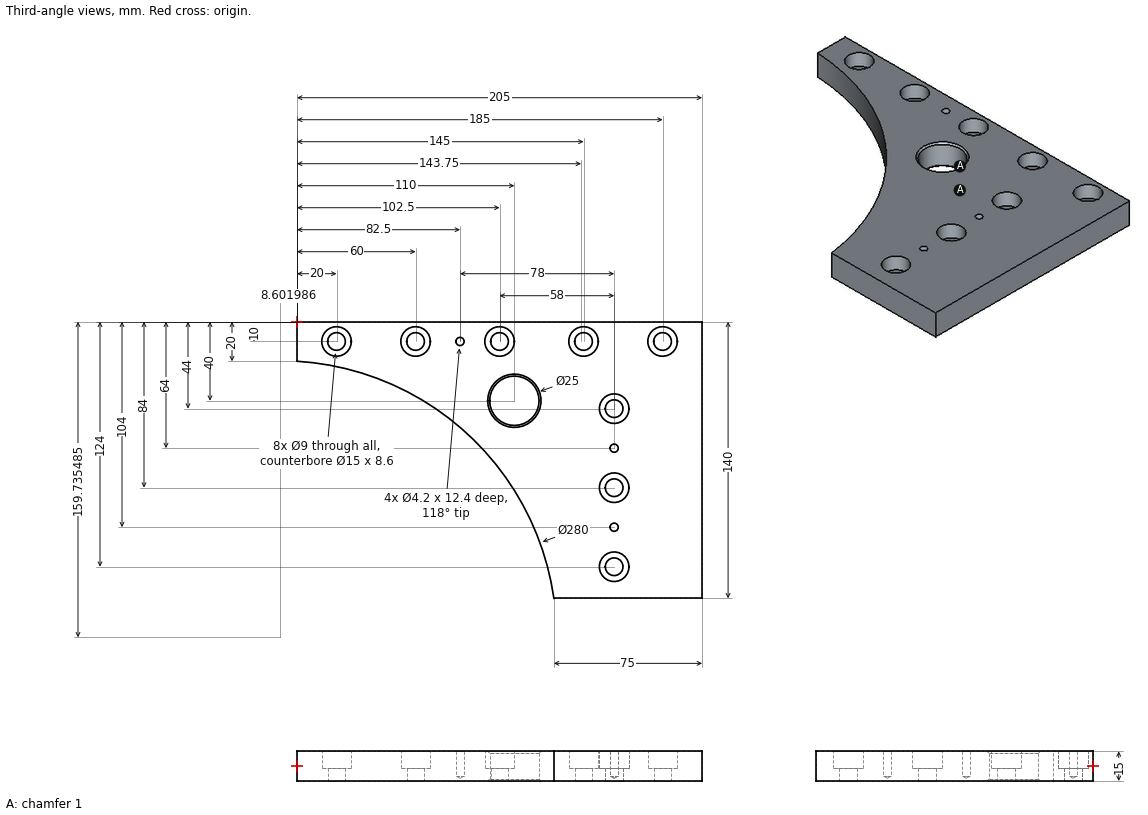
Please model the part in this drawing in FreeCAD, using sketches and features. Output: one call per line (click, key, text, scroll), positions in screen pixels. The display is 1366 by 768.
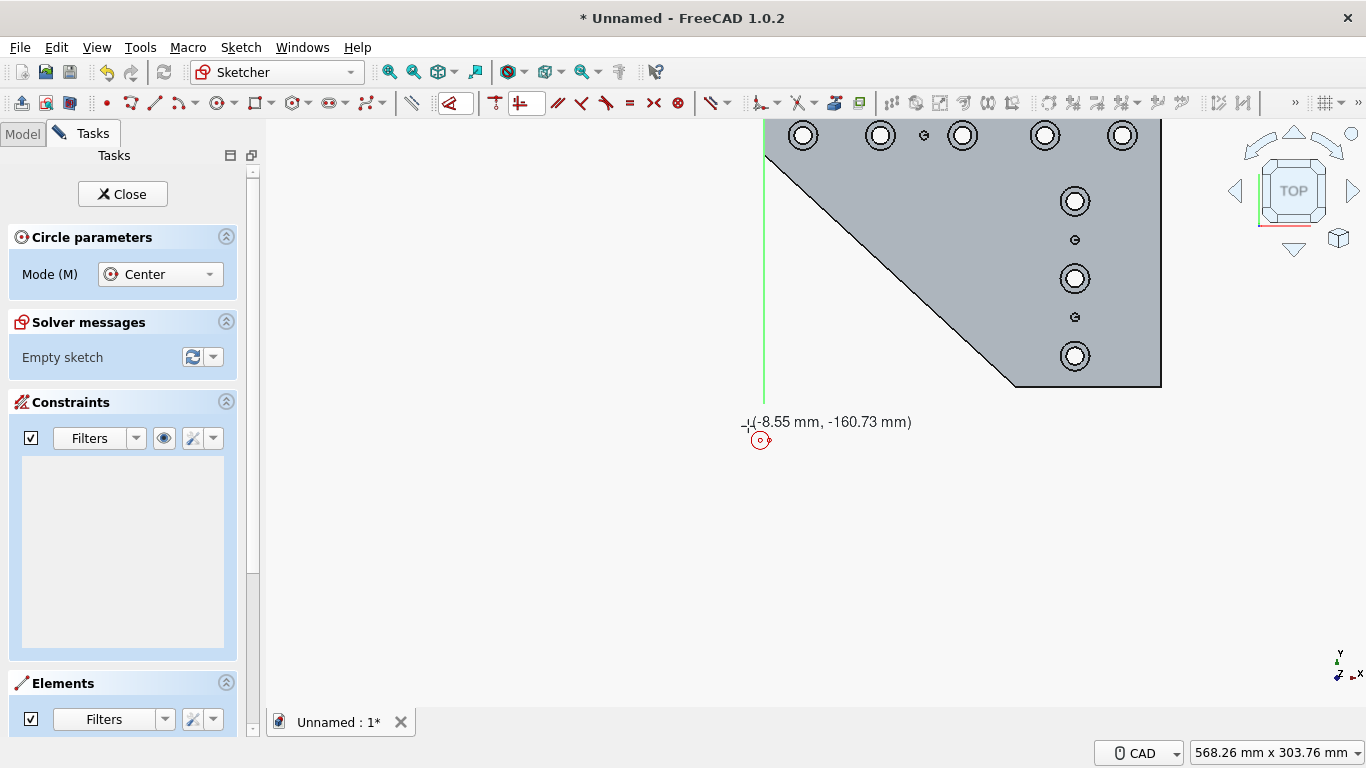
click(748, 425)
click(939, 234)
key(Escape)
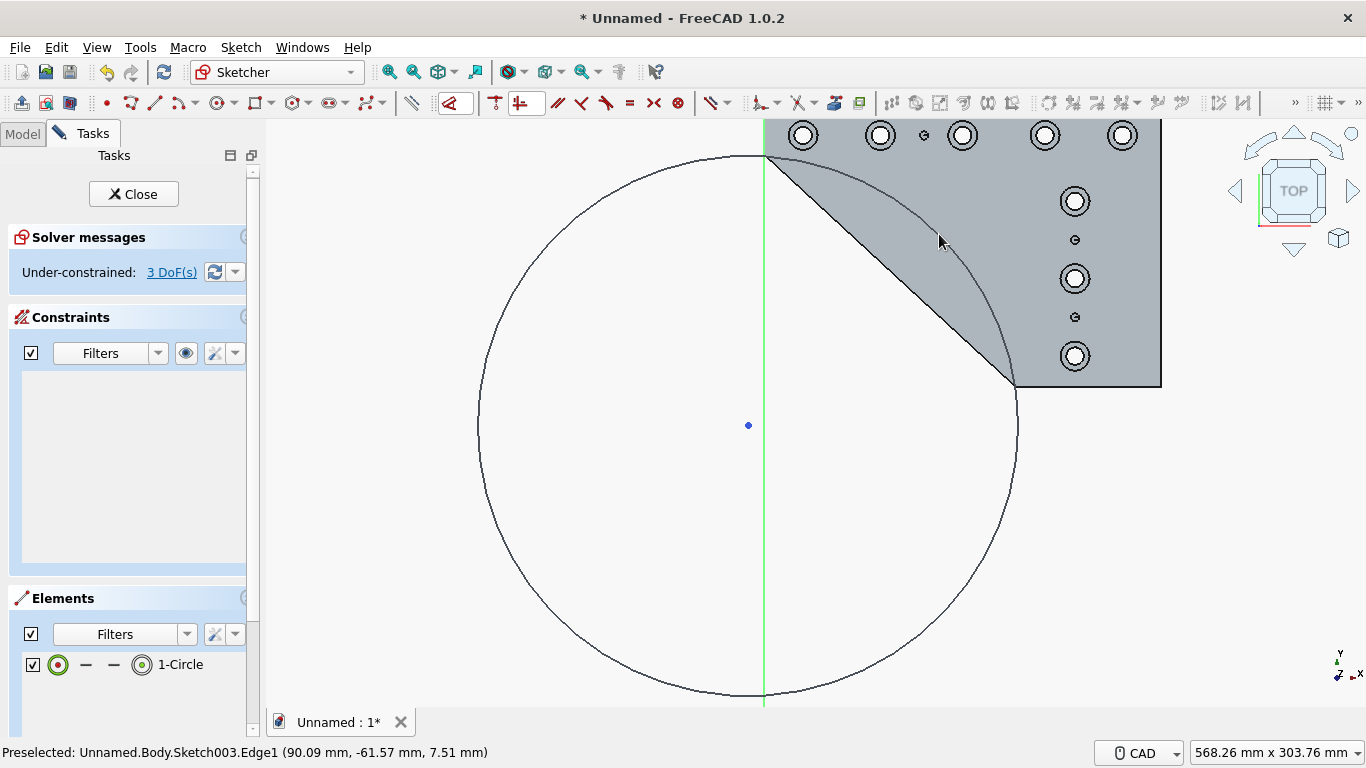
click(938, 234)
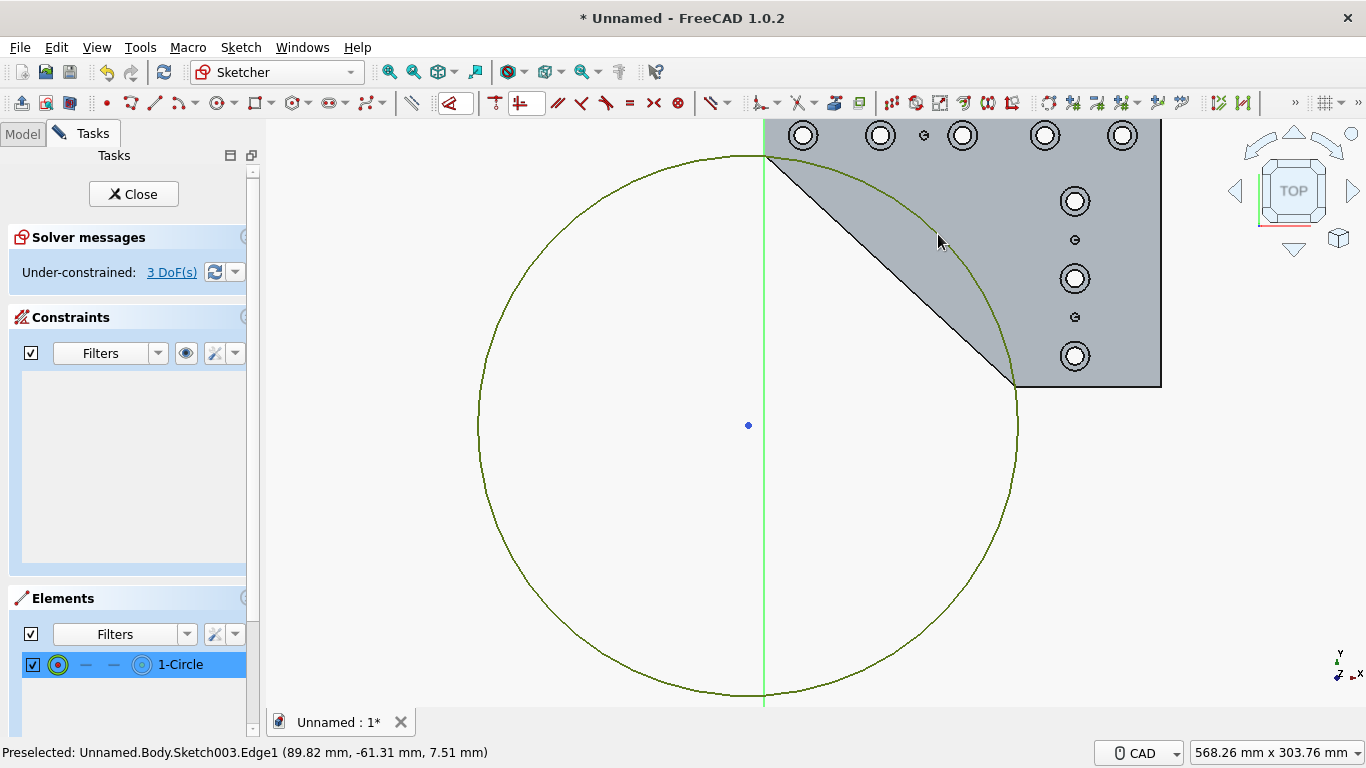
key(k)
key(o)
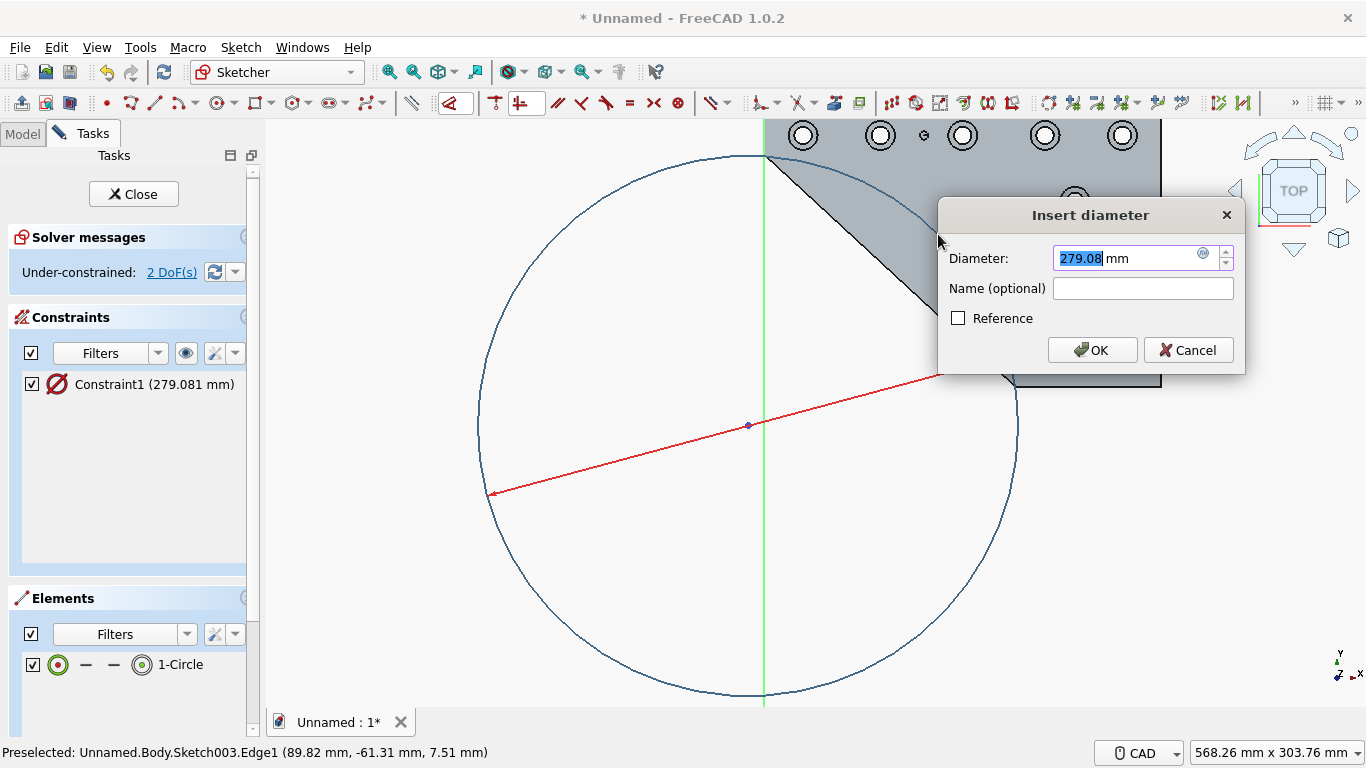
text(280)
key(Return)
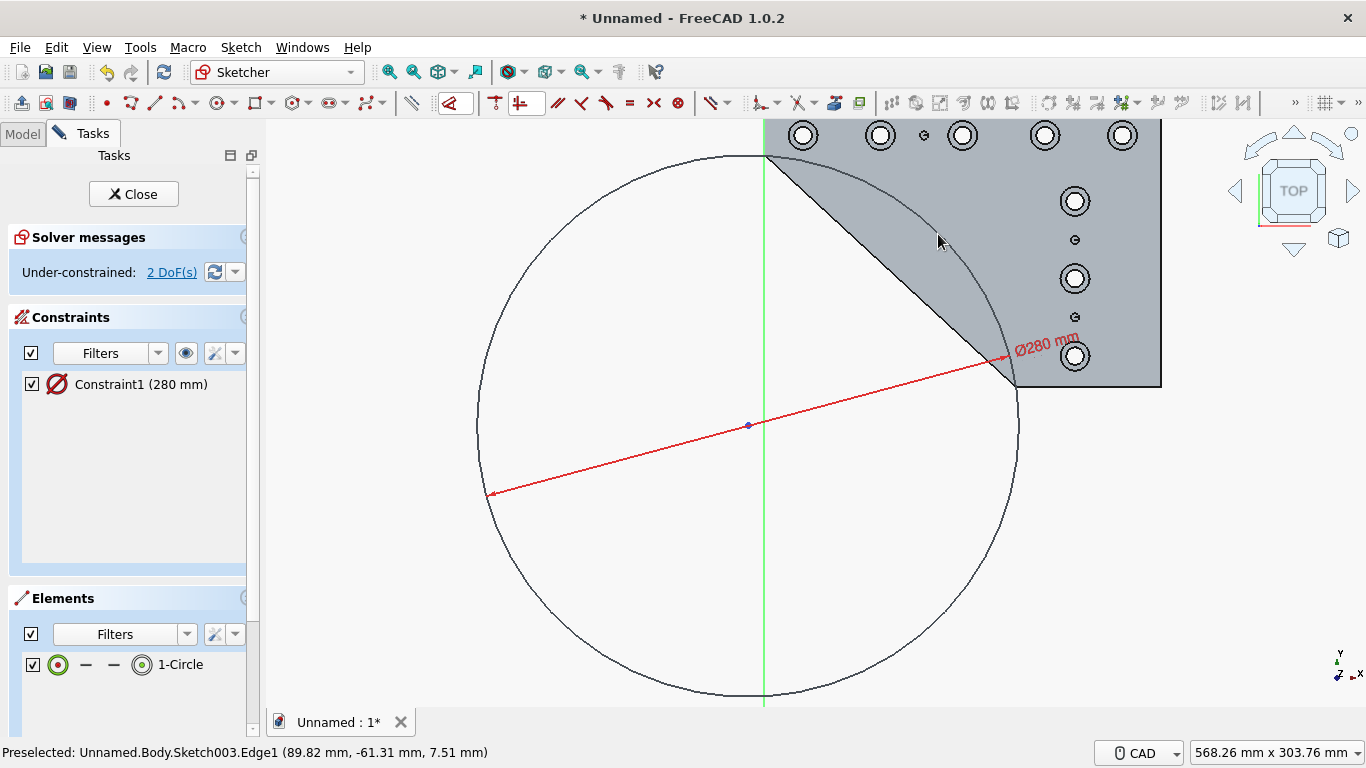
scroll(748, 426, up, 5)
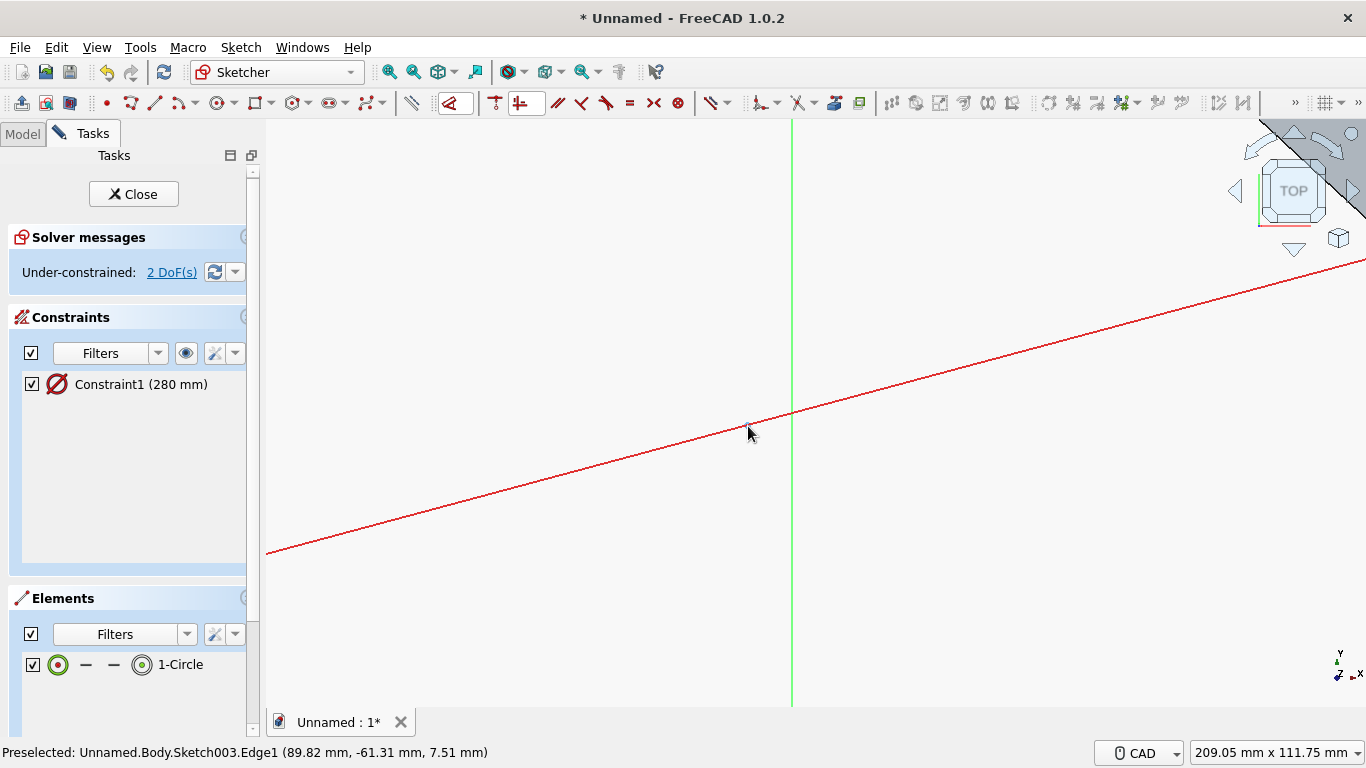
click(747, 425)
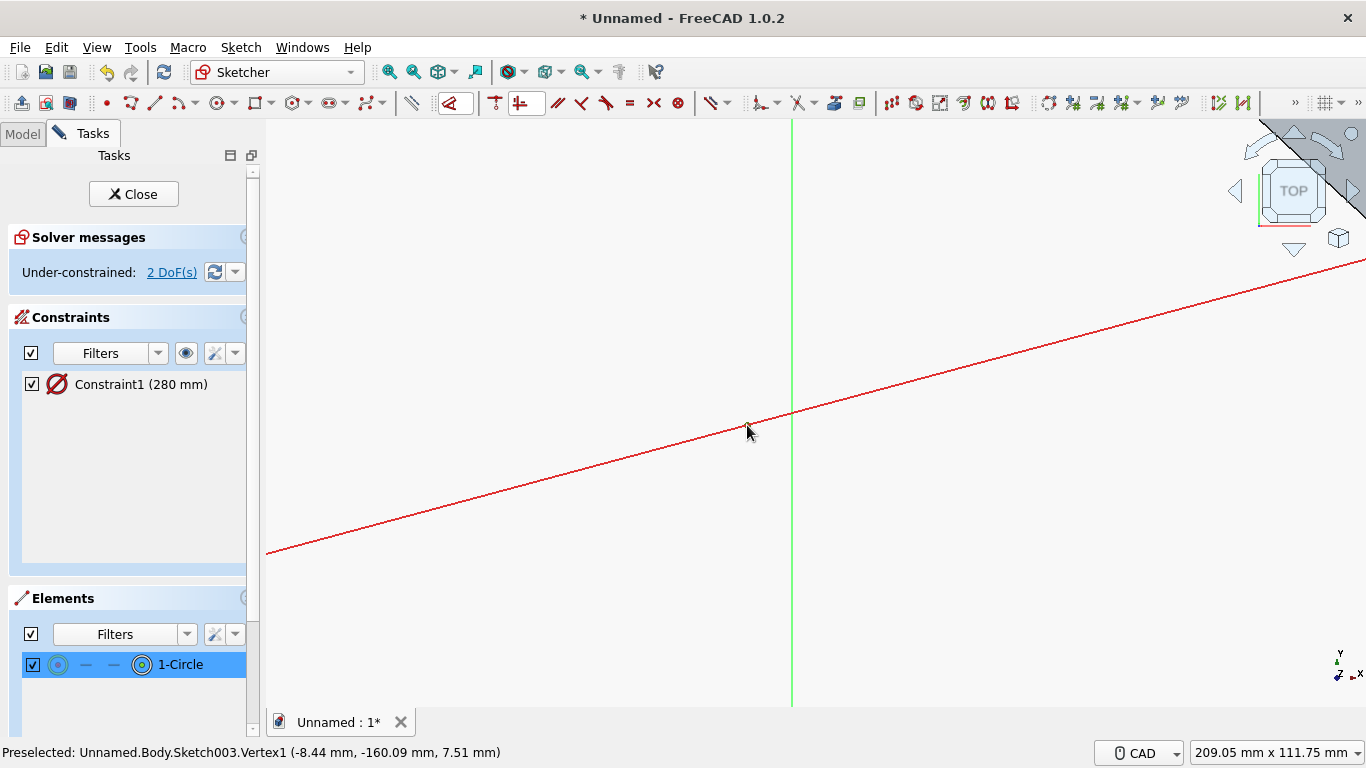
click(468, 104)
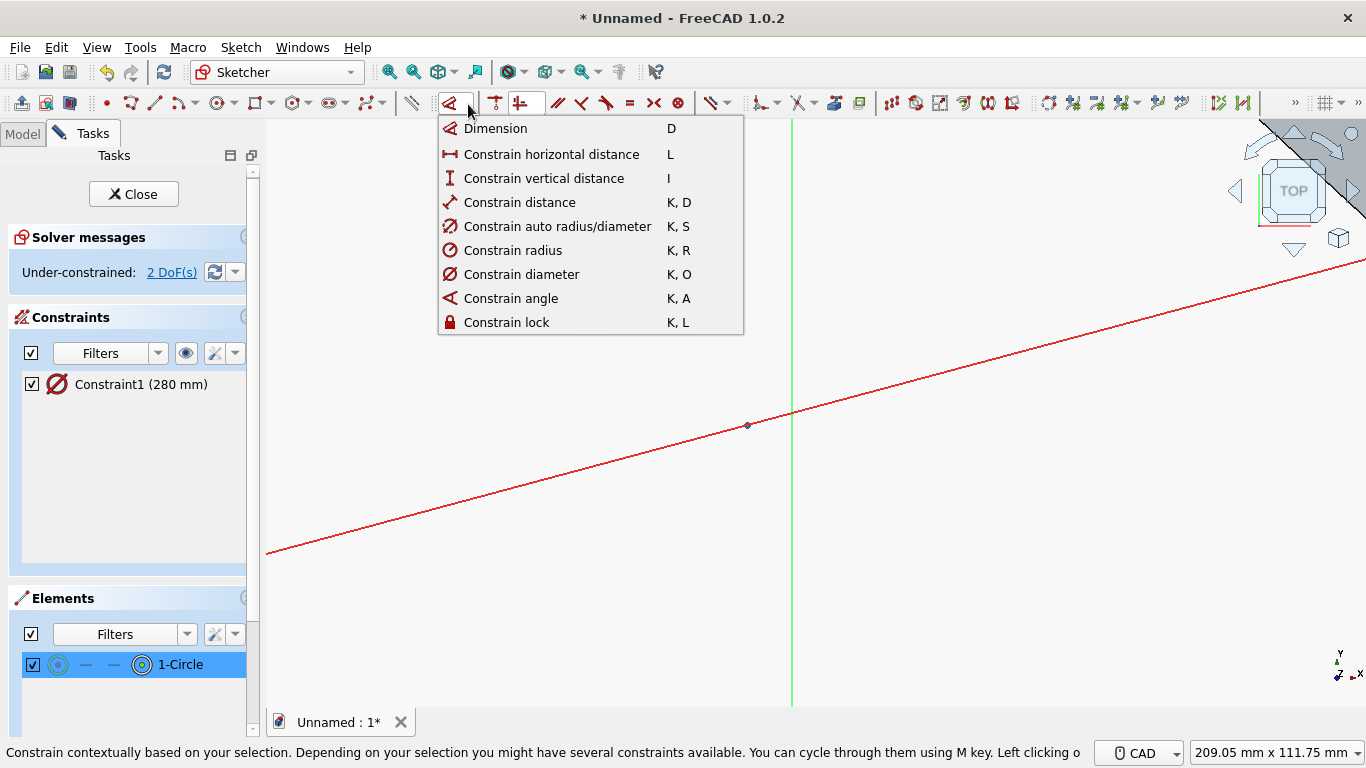
click(591, 154)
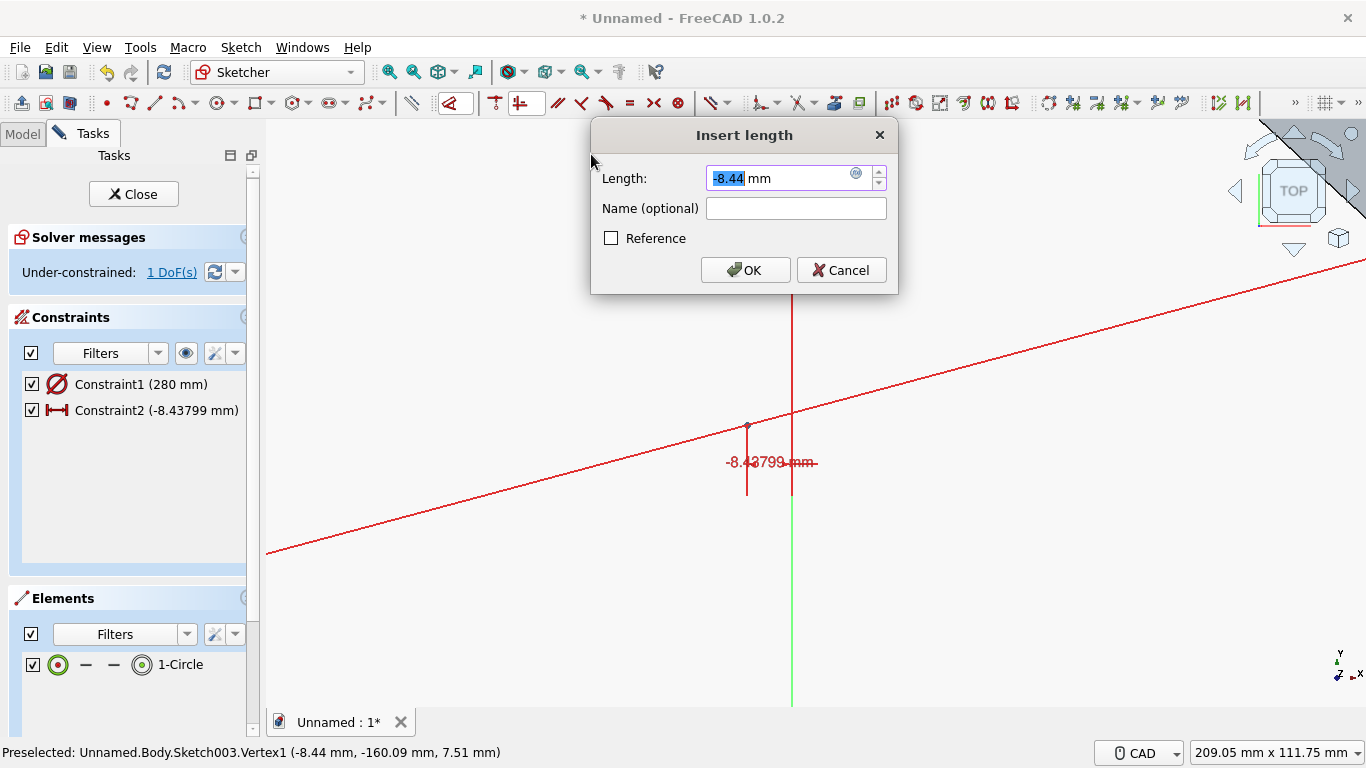
text(-8.601986)
key(Return)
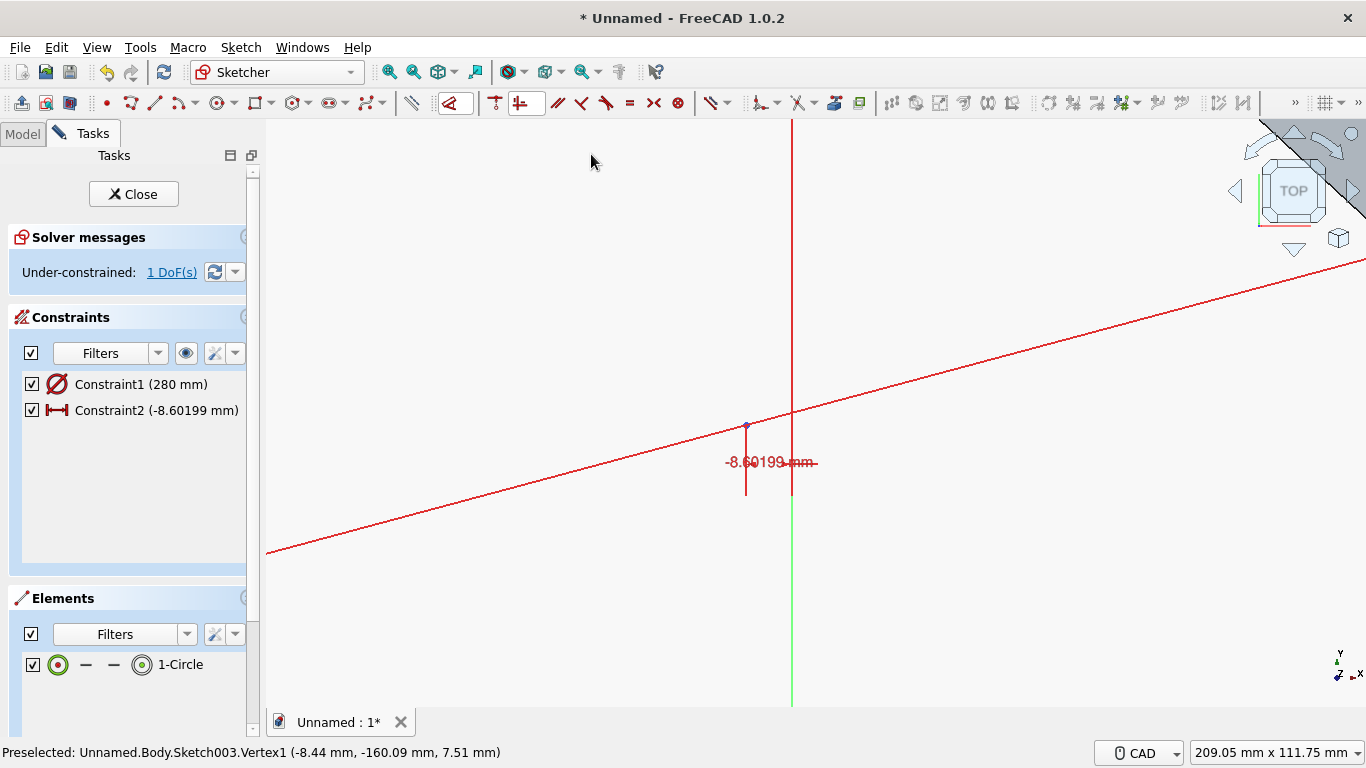
scroll(748, 427, down, 7)